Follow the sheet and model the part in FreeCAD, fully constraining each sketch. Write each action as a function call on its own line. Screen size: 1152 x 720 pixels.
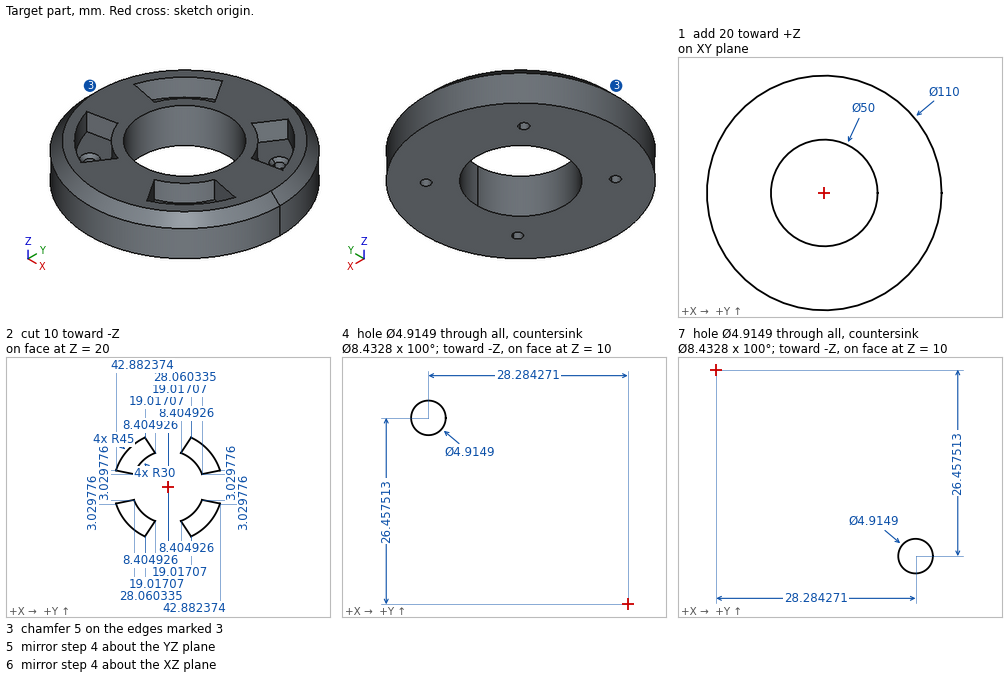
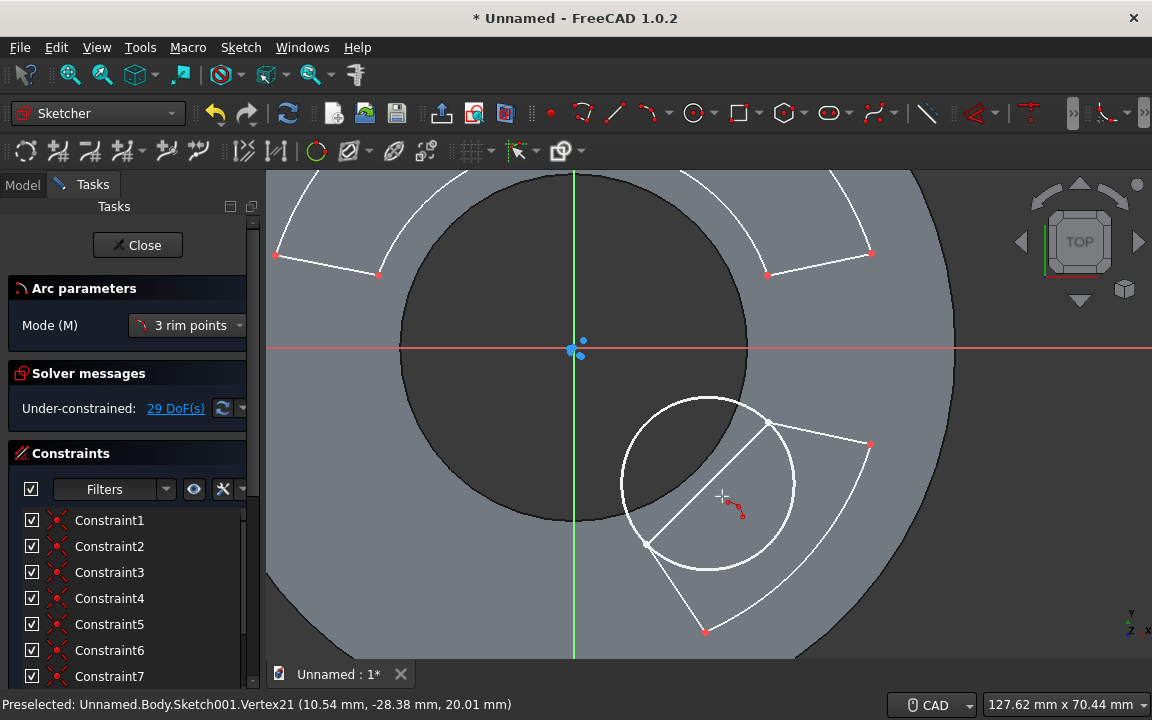
click(721, 495)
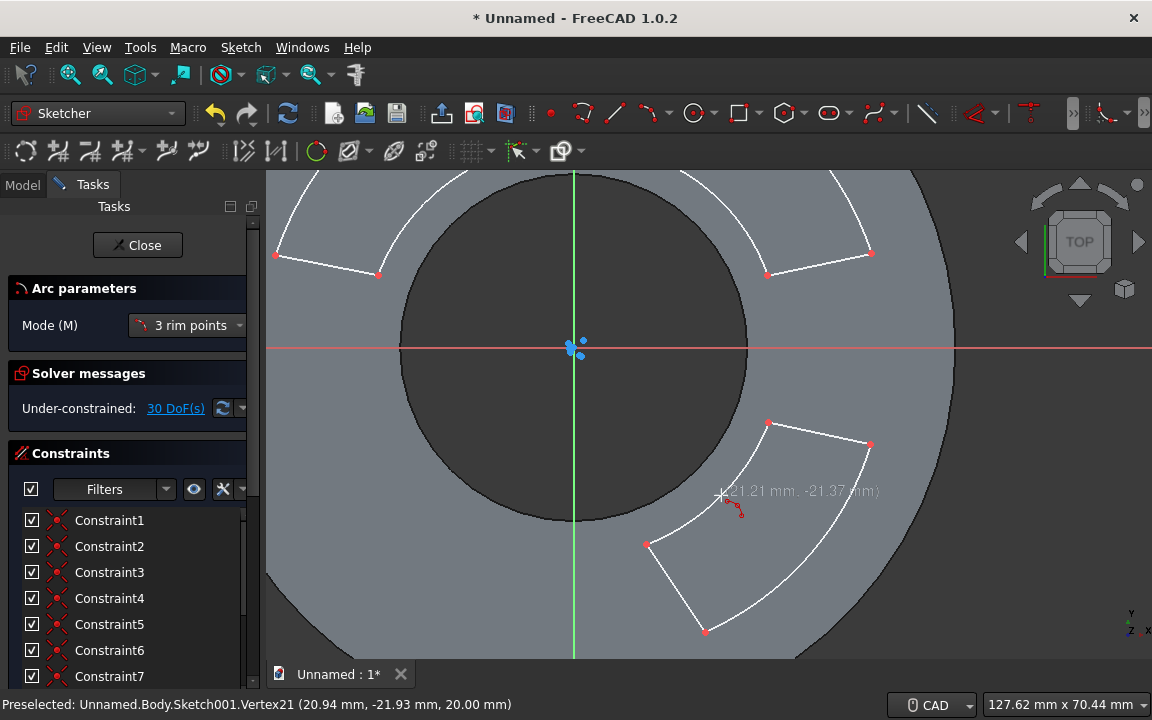
click(616, 114)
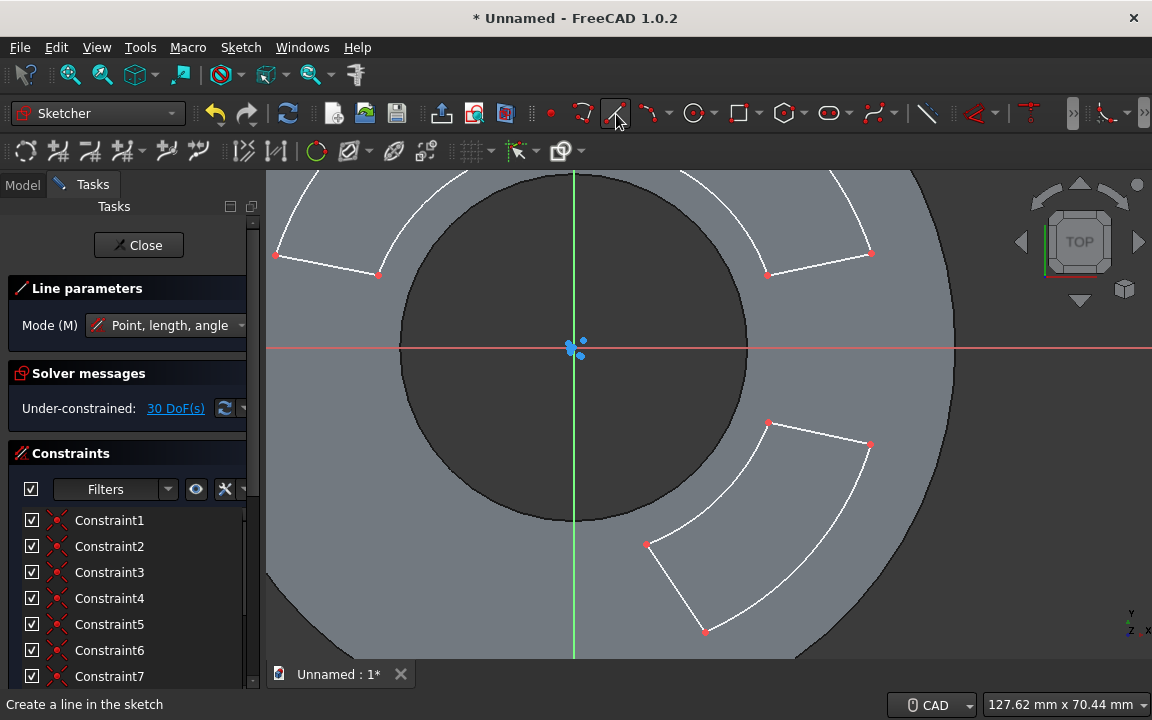
click(379, 421)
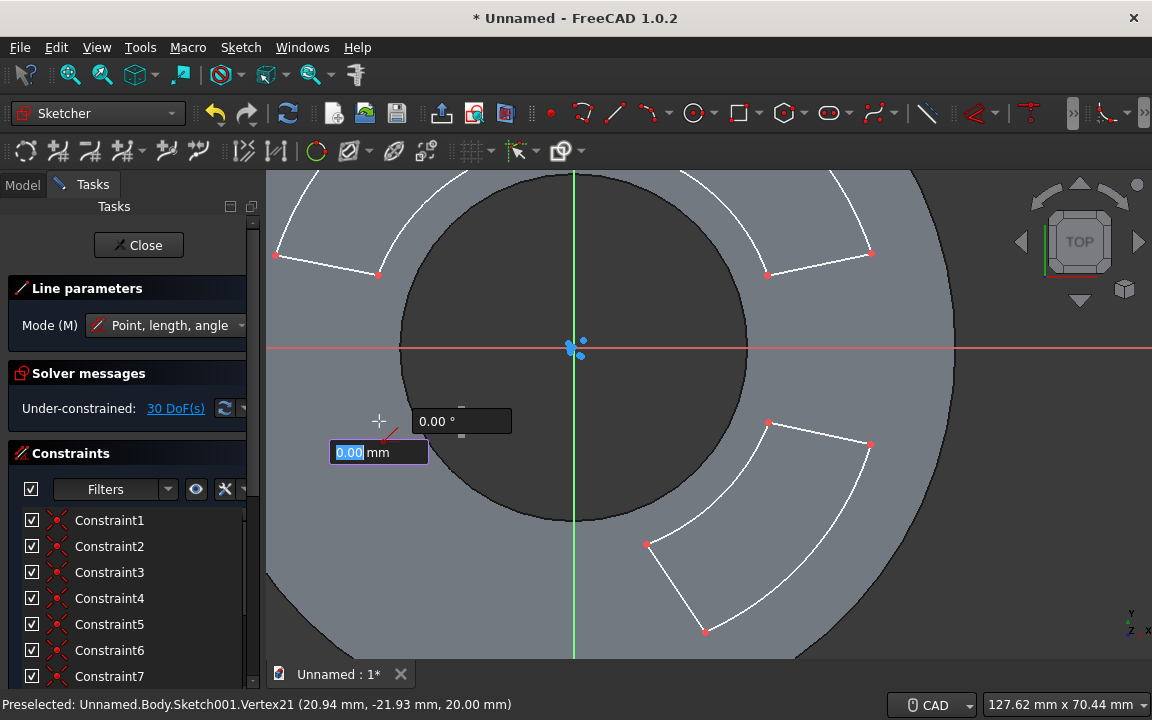
scroll(722, 496, down, 3)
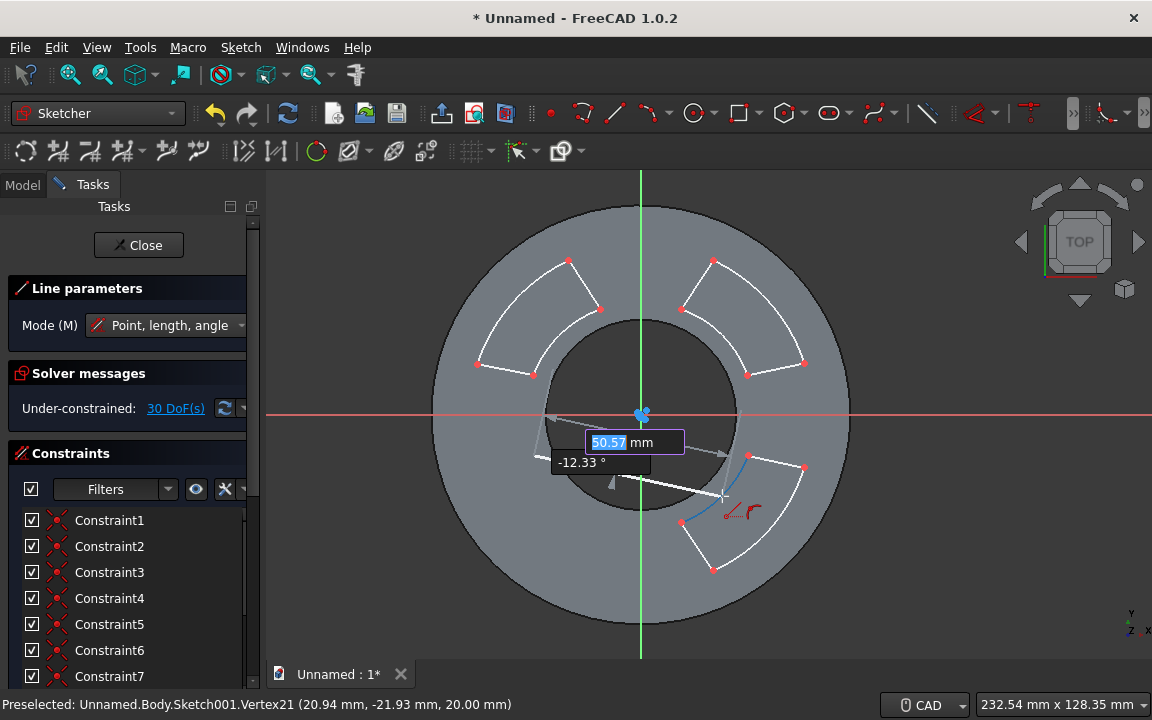
click(477, 467)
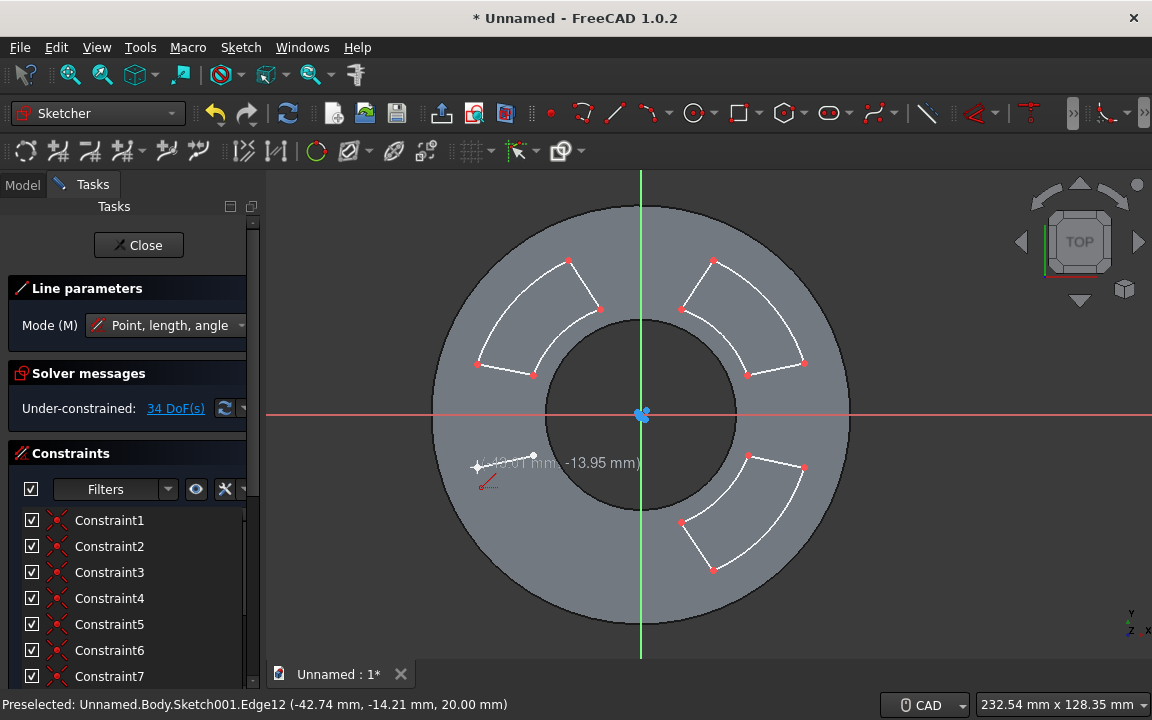
click(568, 570)
click(600, 522)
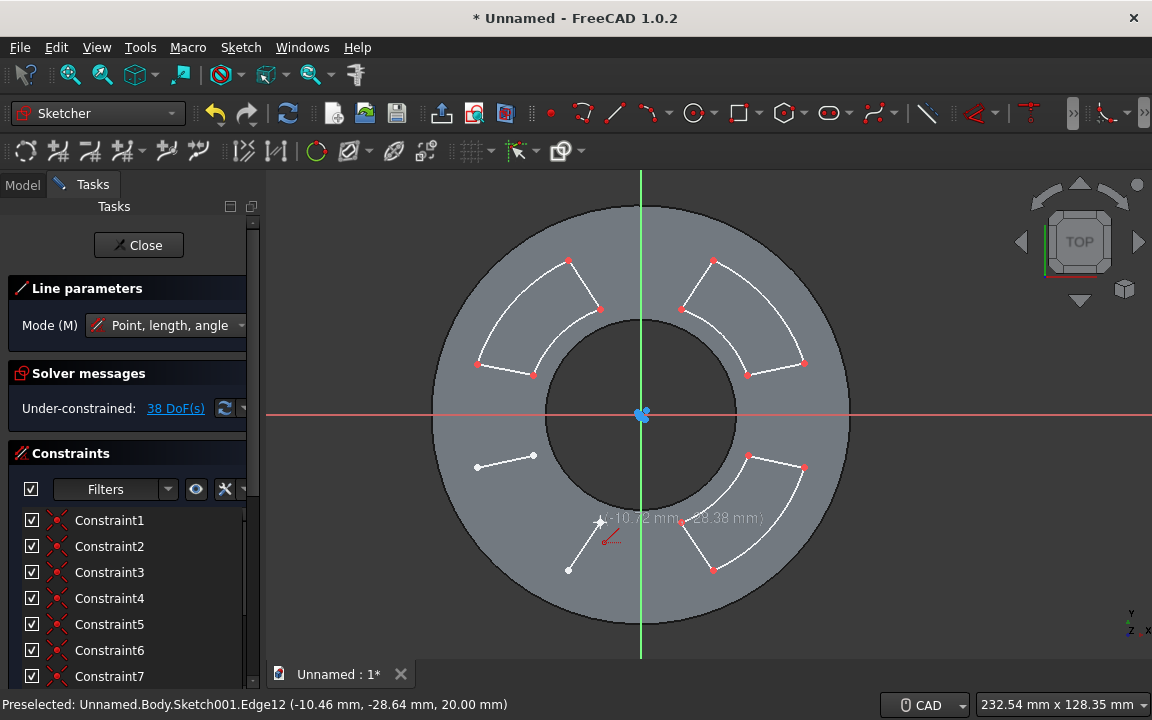
click(648, 114)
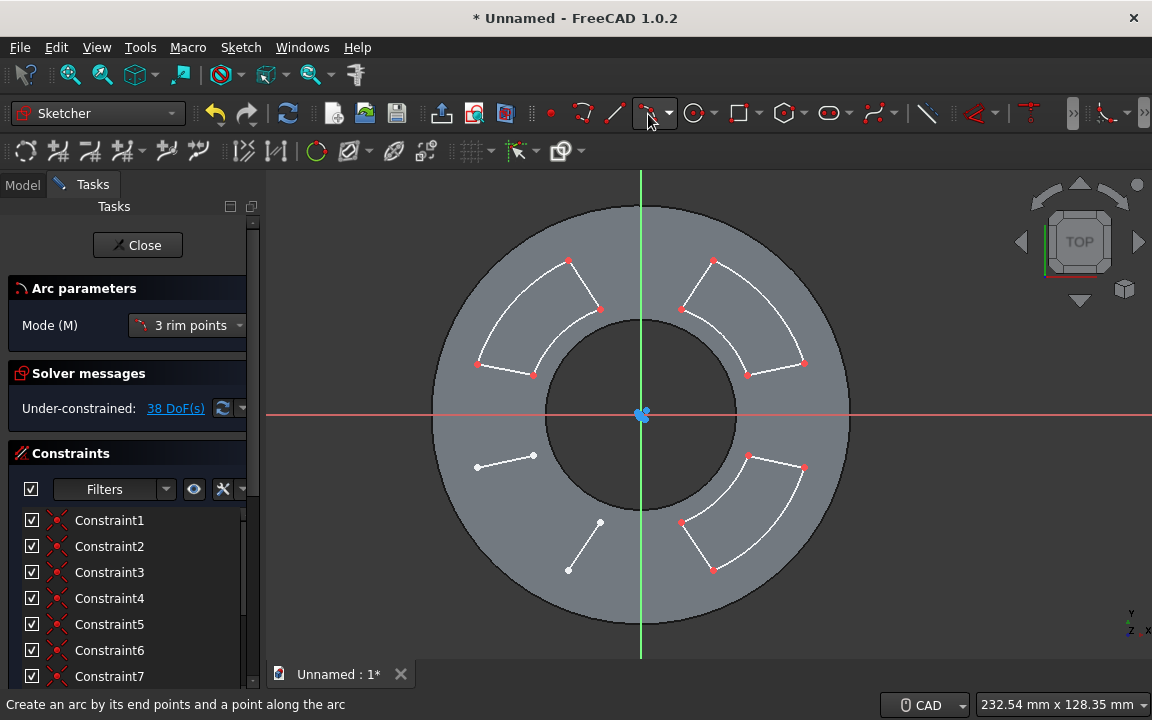
click(477, 468)
click(568, 571)
click(512, 528)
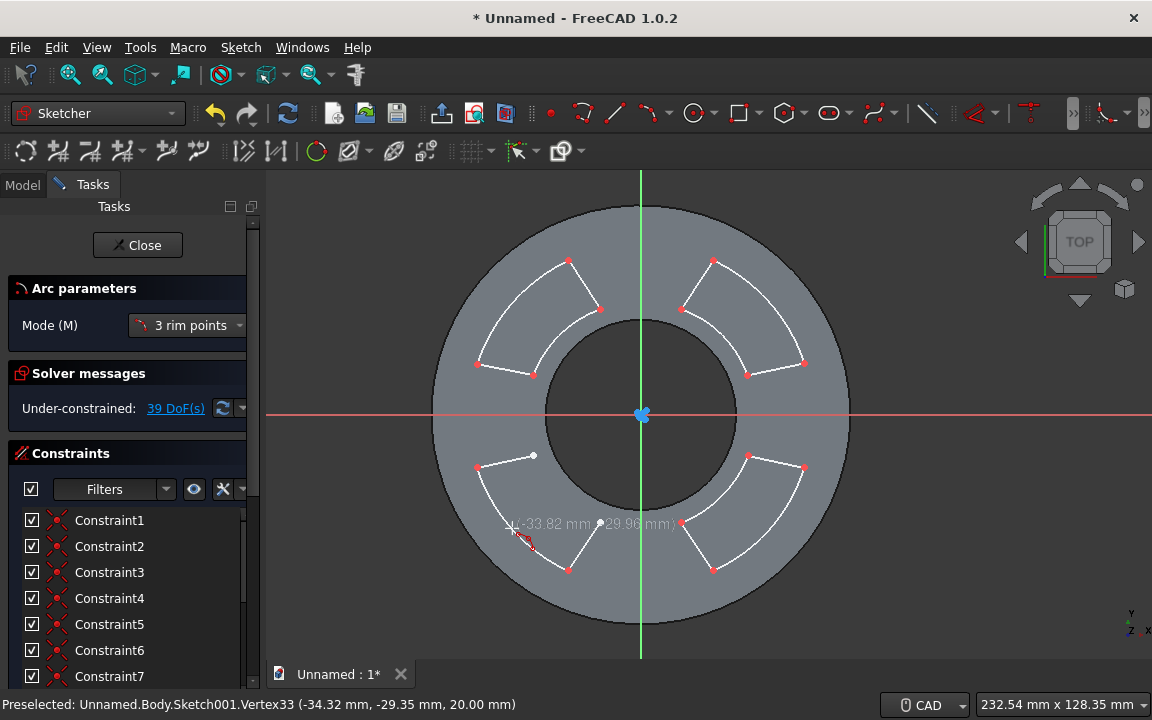
click(600, 523)
click(534, 456)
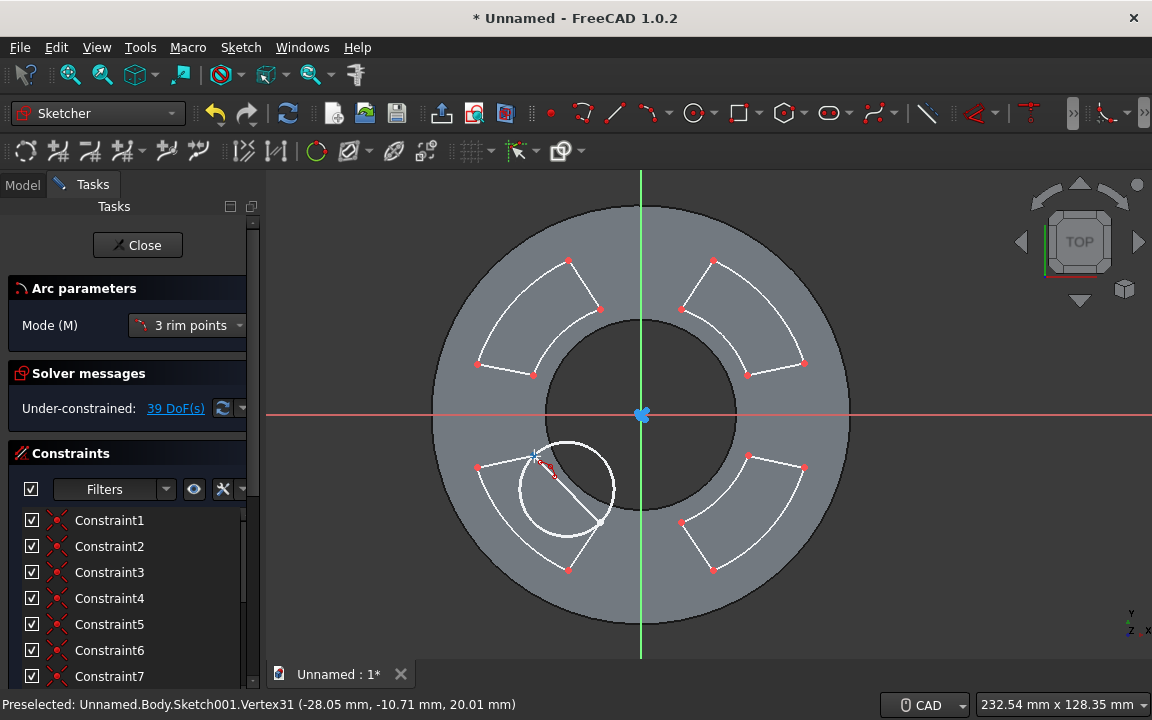
scroll(560, 496, up, 3)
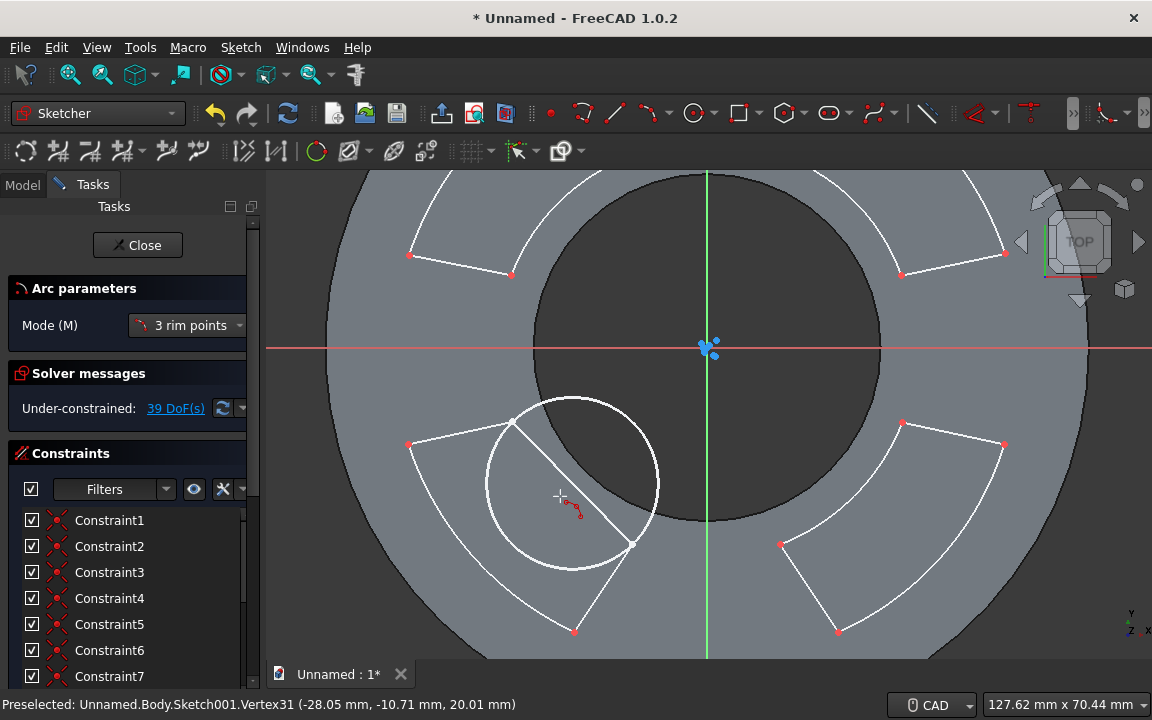
click(560, 495)
key(Escape)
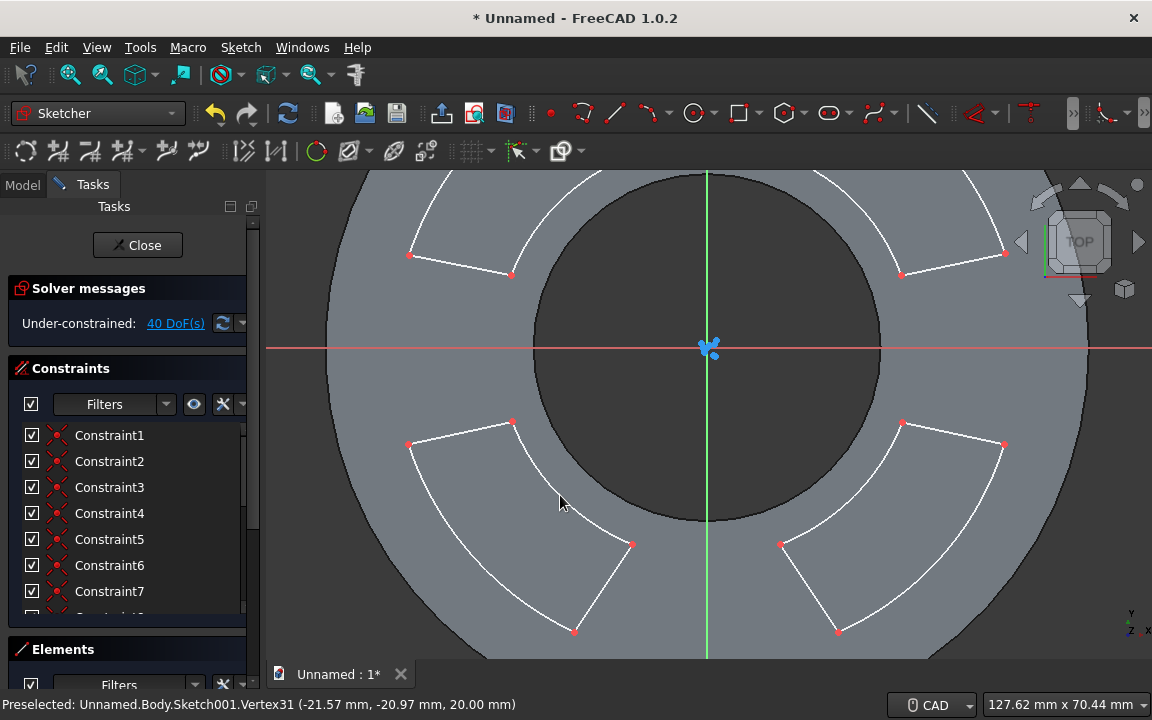
click(429, 208)